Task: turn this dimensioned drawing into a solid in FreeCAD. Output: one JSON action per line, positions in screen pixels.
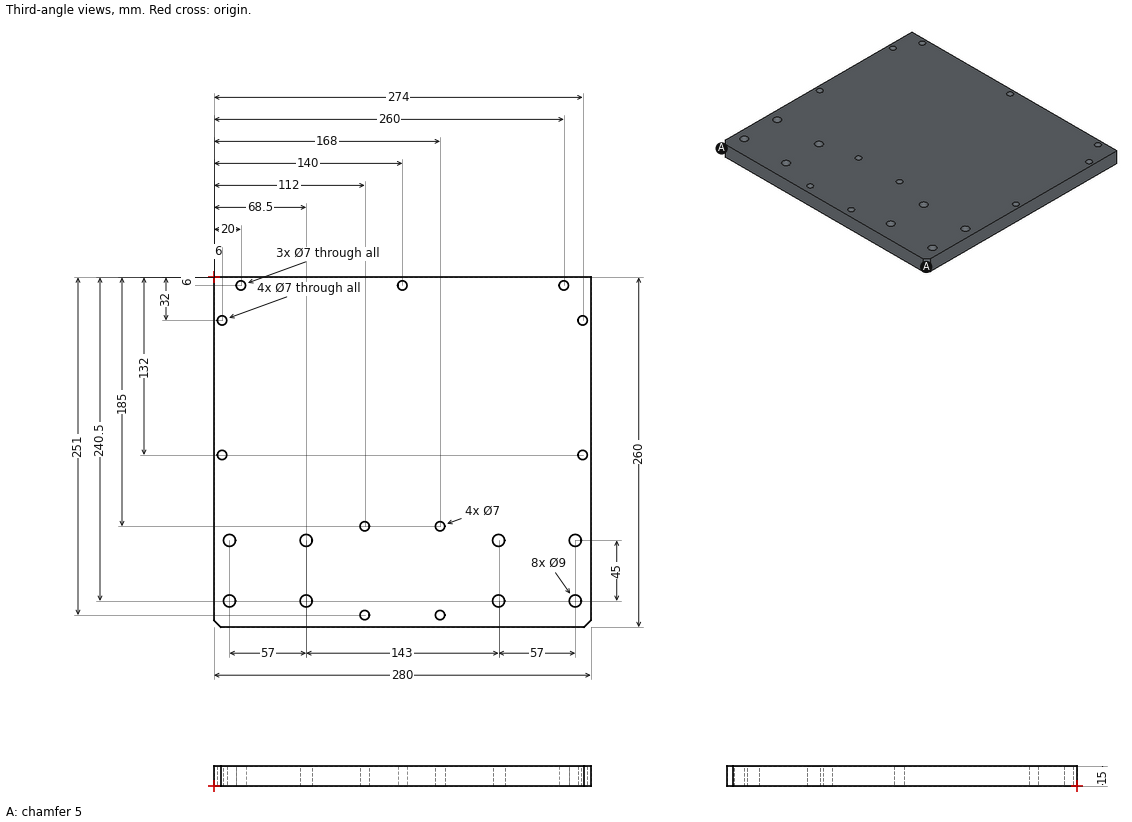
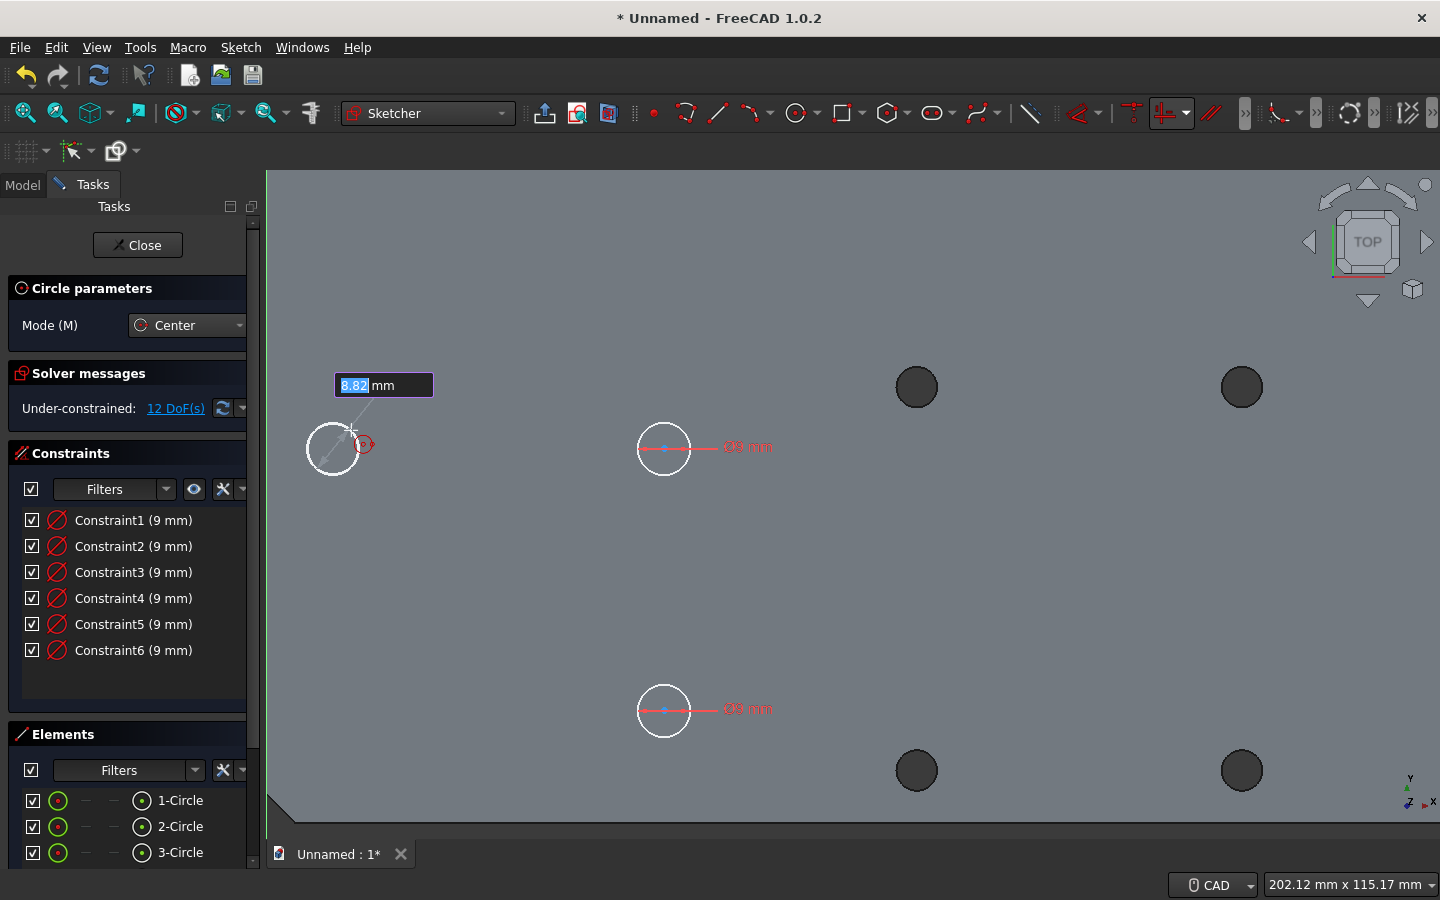
{"action": "type", "text": "9"}
{"action": "key", "text": "Return"}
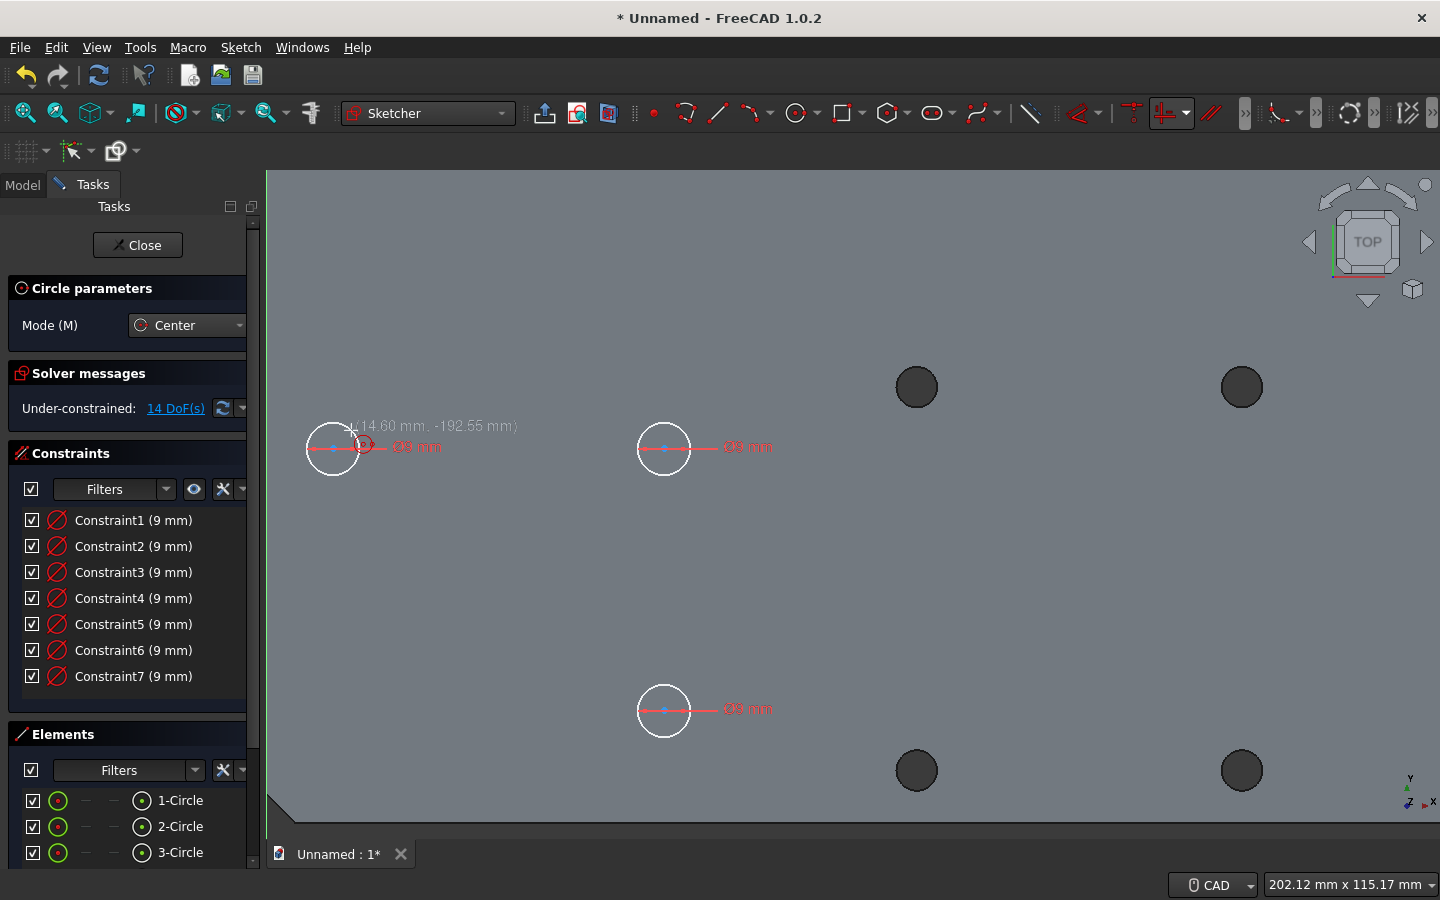
{"action": "left_click", "coordinate": [333, 710]}
{"action": "mouse_move", "coordinate": [351, 691]}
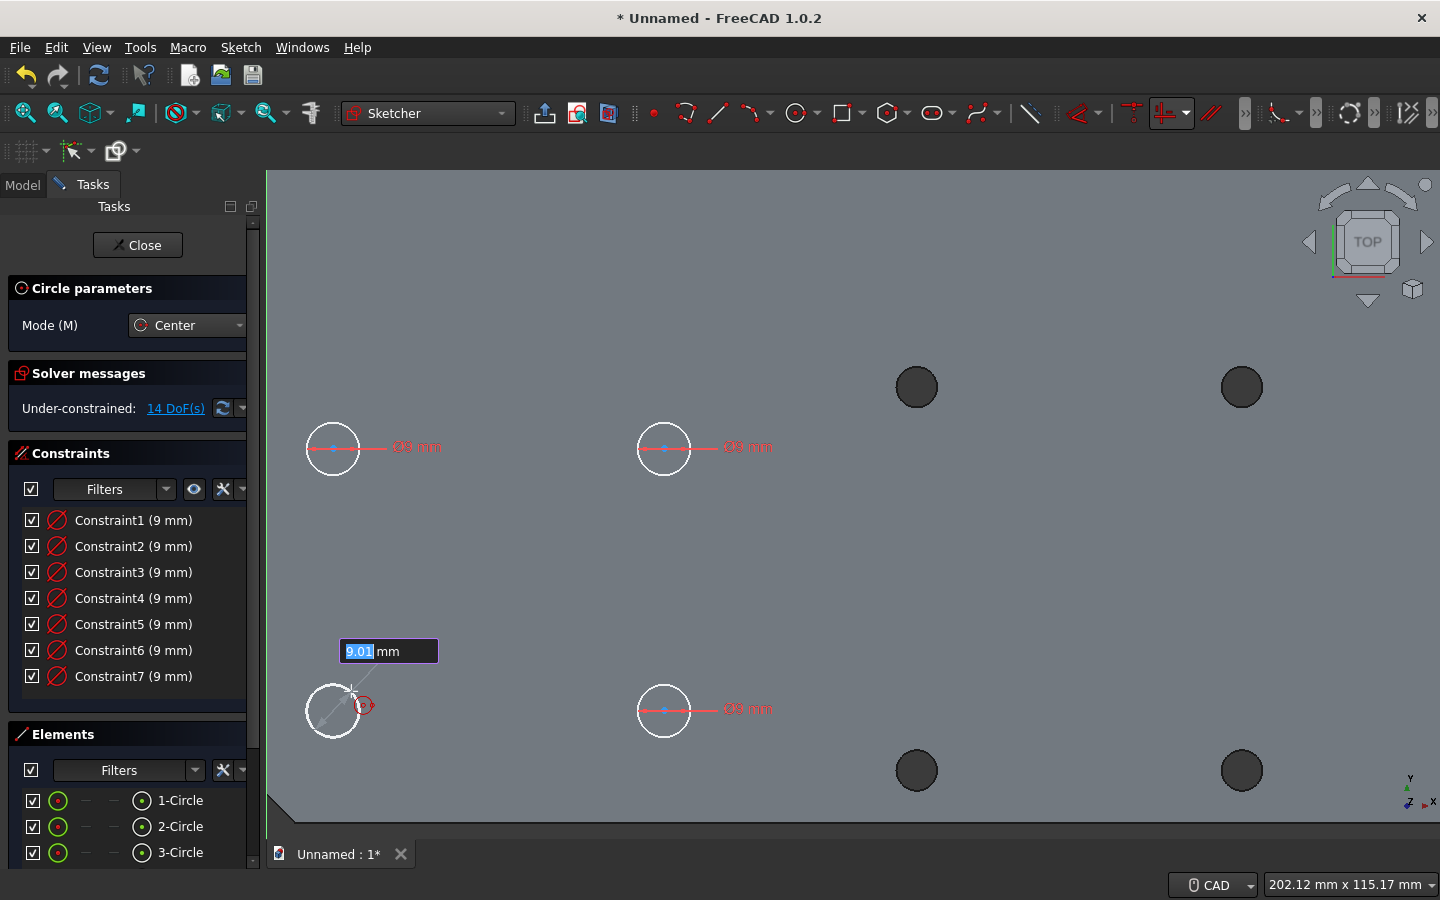
{"action": "type", "text": "9"}
{"action": "key", "text": "Return"}
{"action": "key", "text": "Escape"}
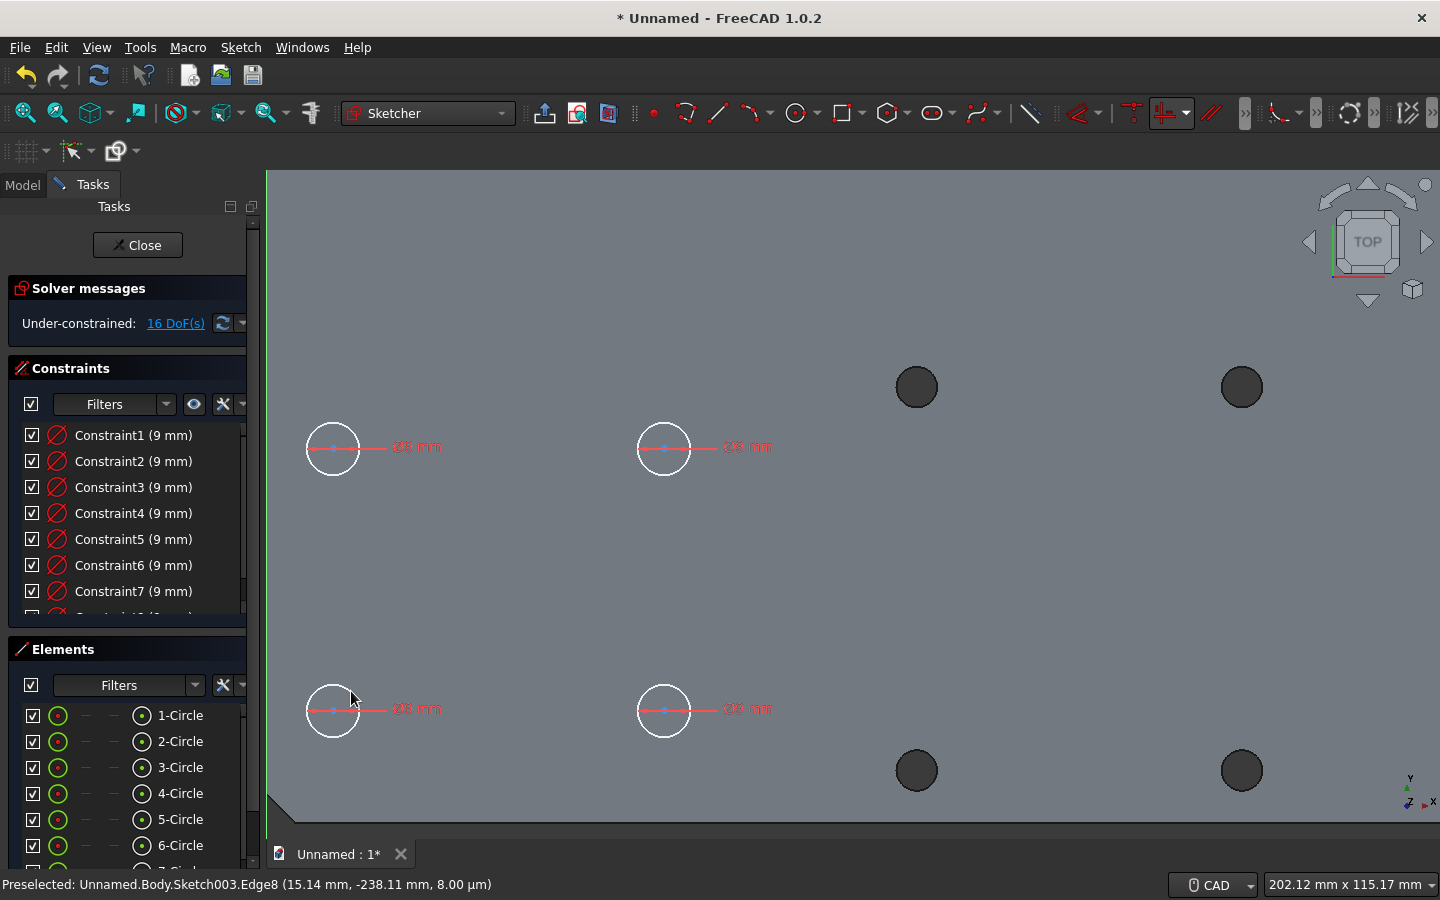
{"action": "scroll", "coordinate": [666, 712], "scroll_direction": "down", "scroll_amount": 6}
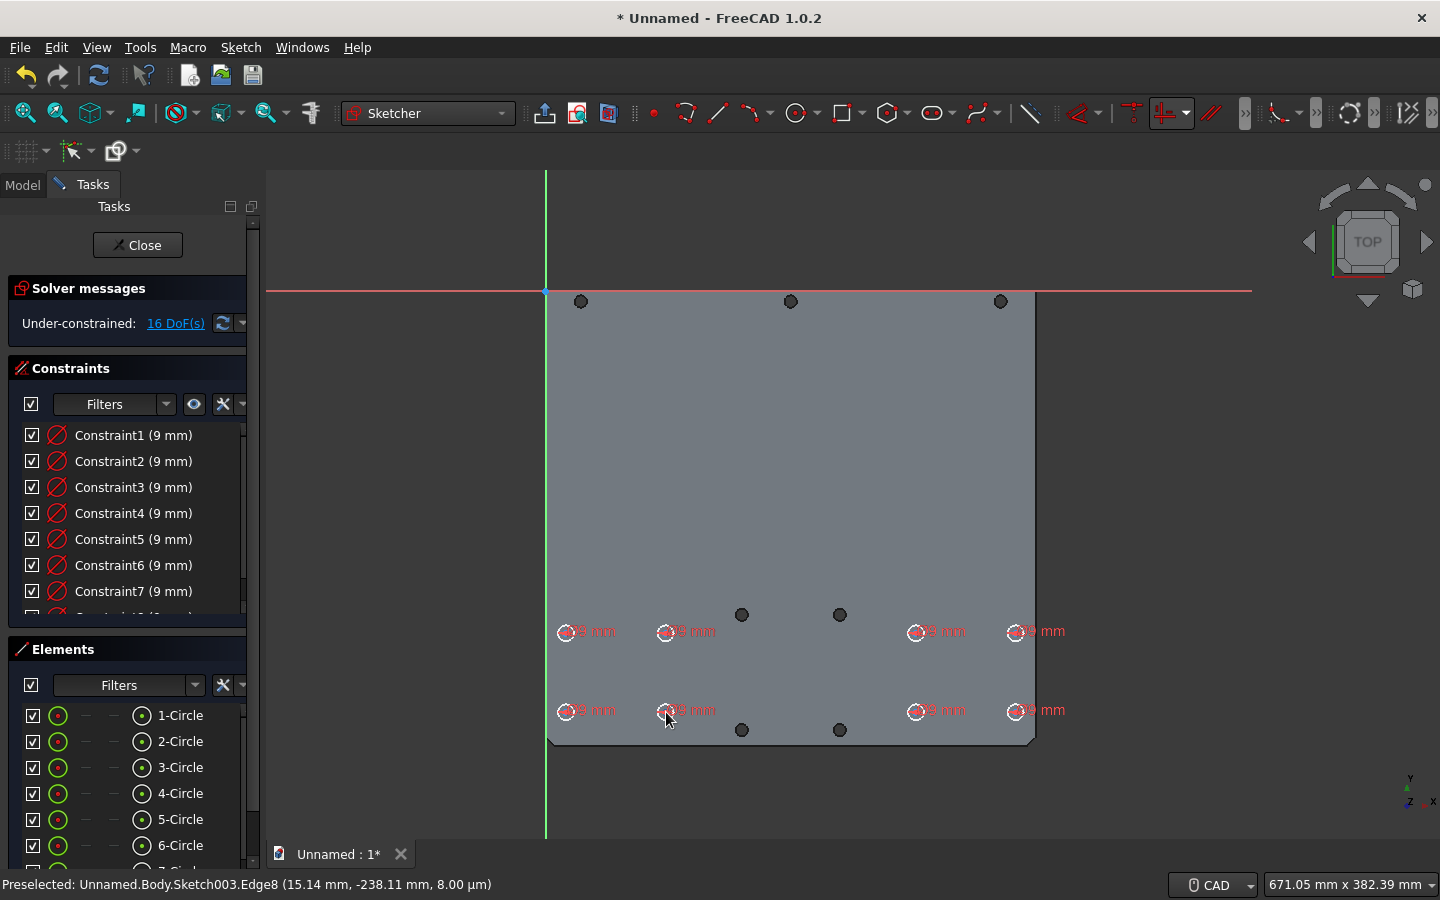
{"action": "left_click", "coordinate": [1016, 712]}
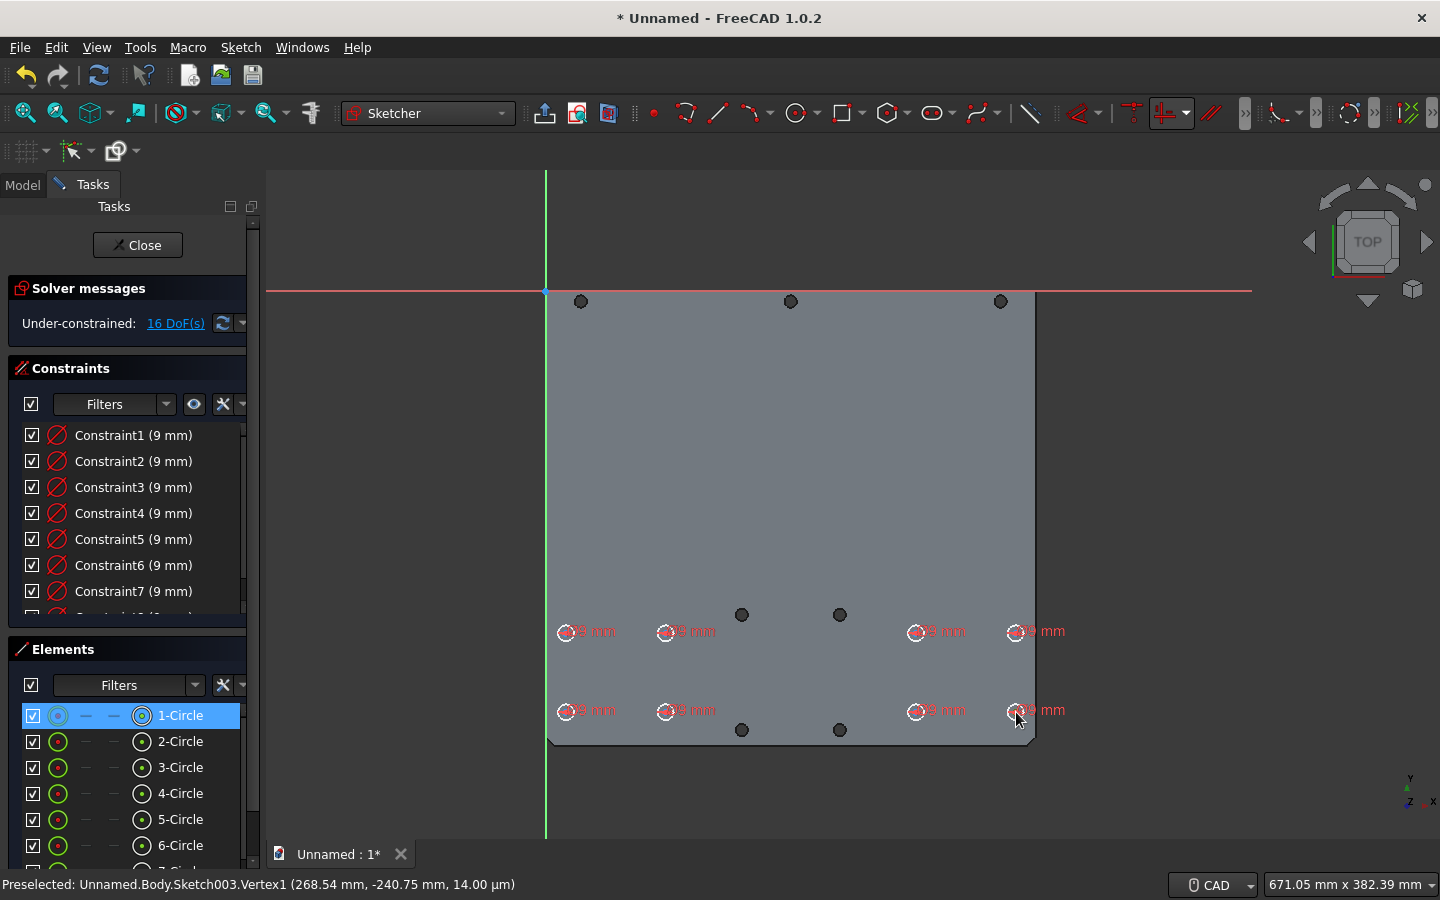
{"action": "left_click", "coordinate": [1016, 633]}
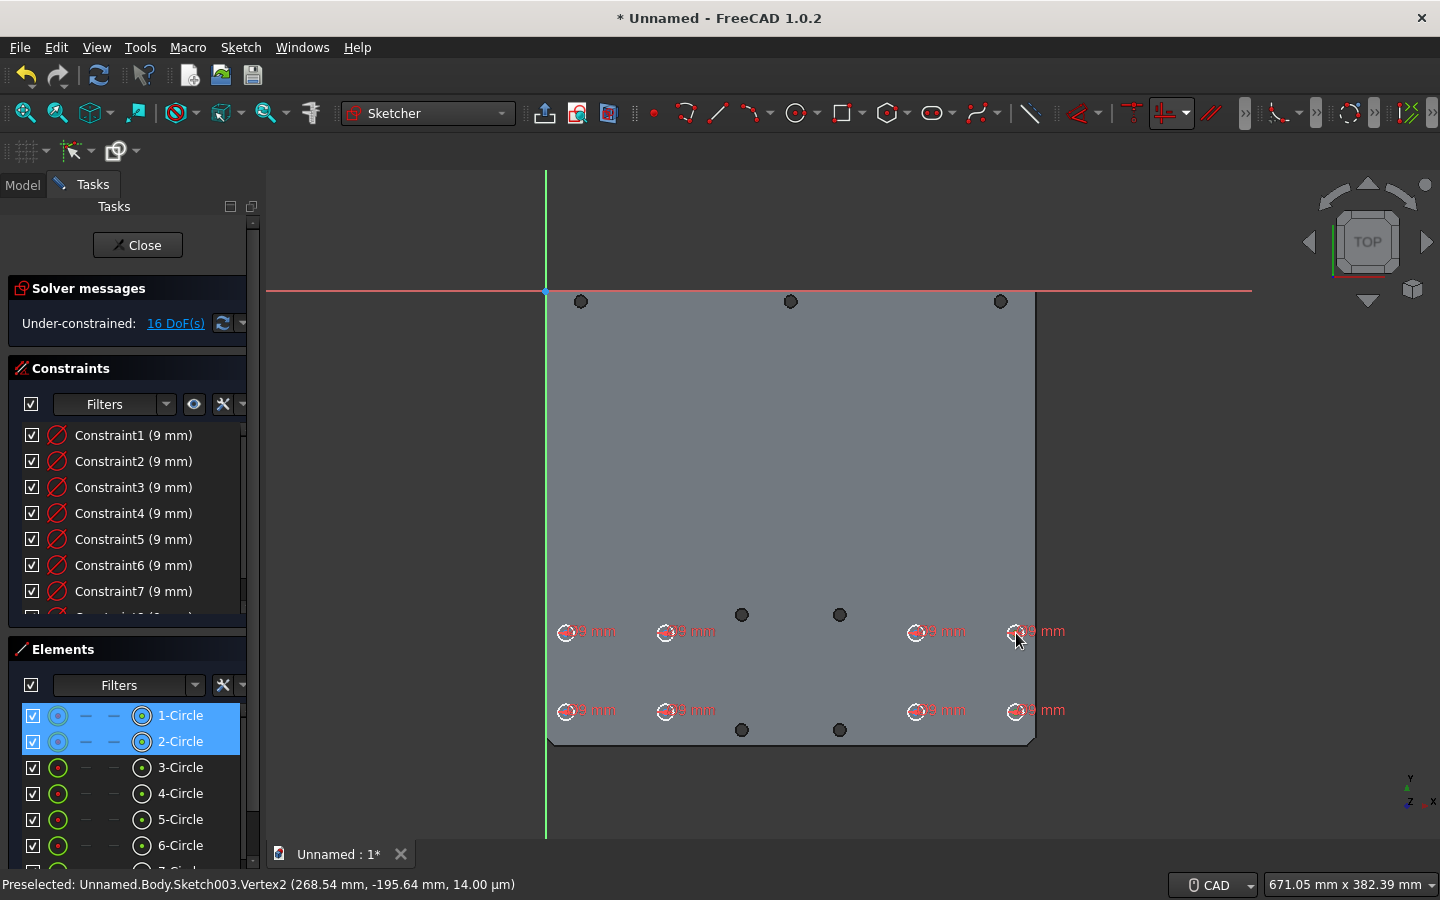
{"action": "key", "text": "v"}